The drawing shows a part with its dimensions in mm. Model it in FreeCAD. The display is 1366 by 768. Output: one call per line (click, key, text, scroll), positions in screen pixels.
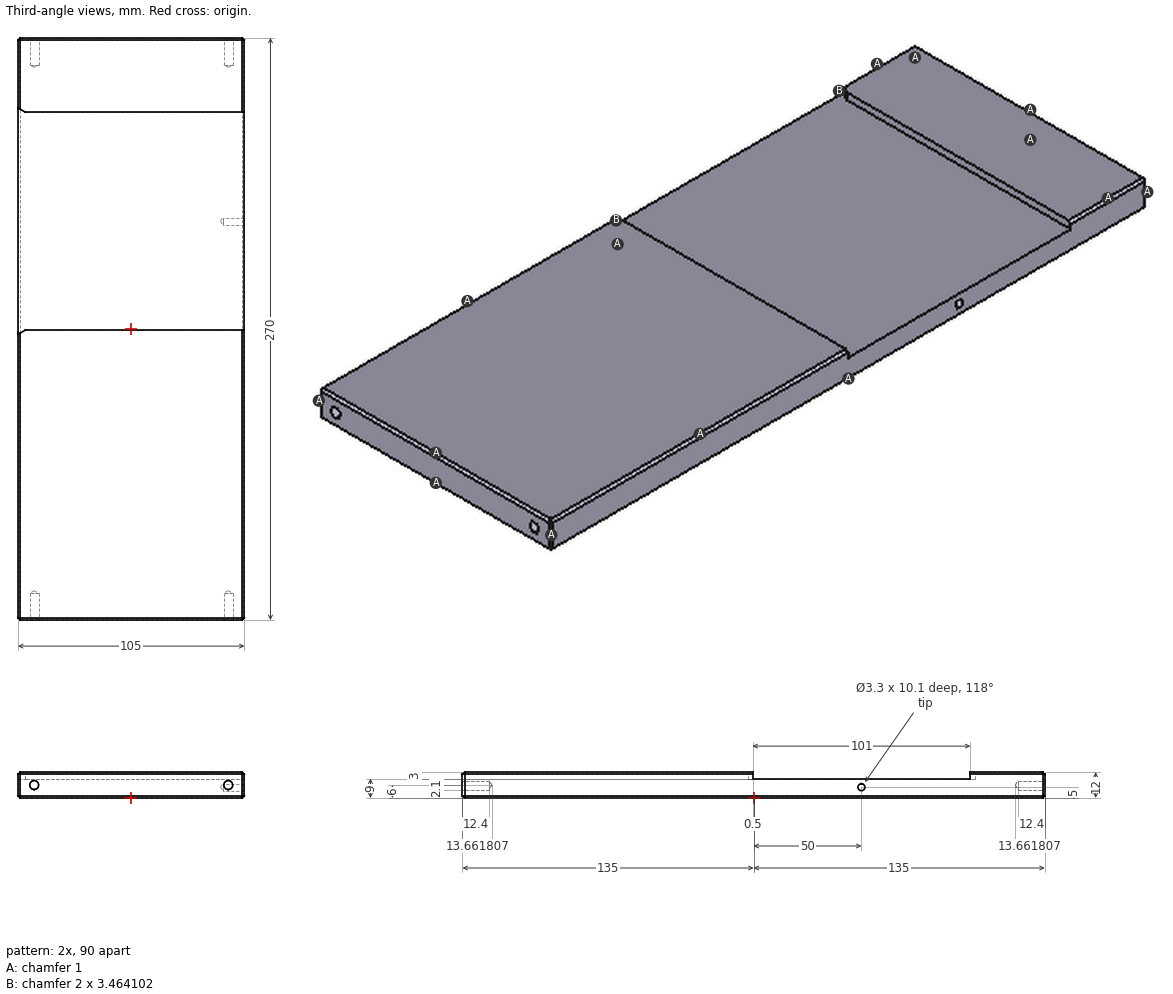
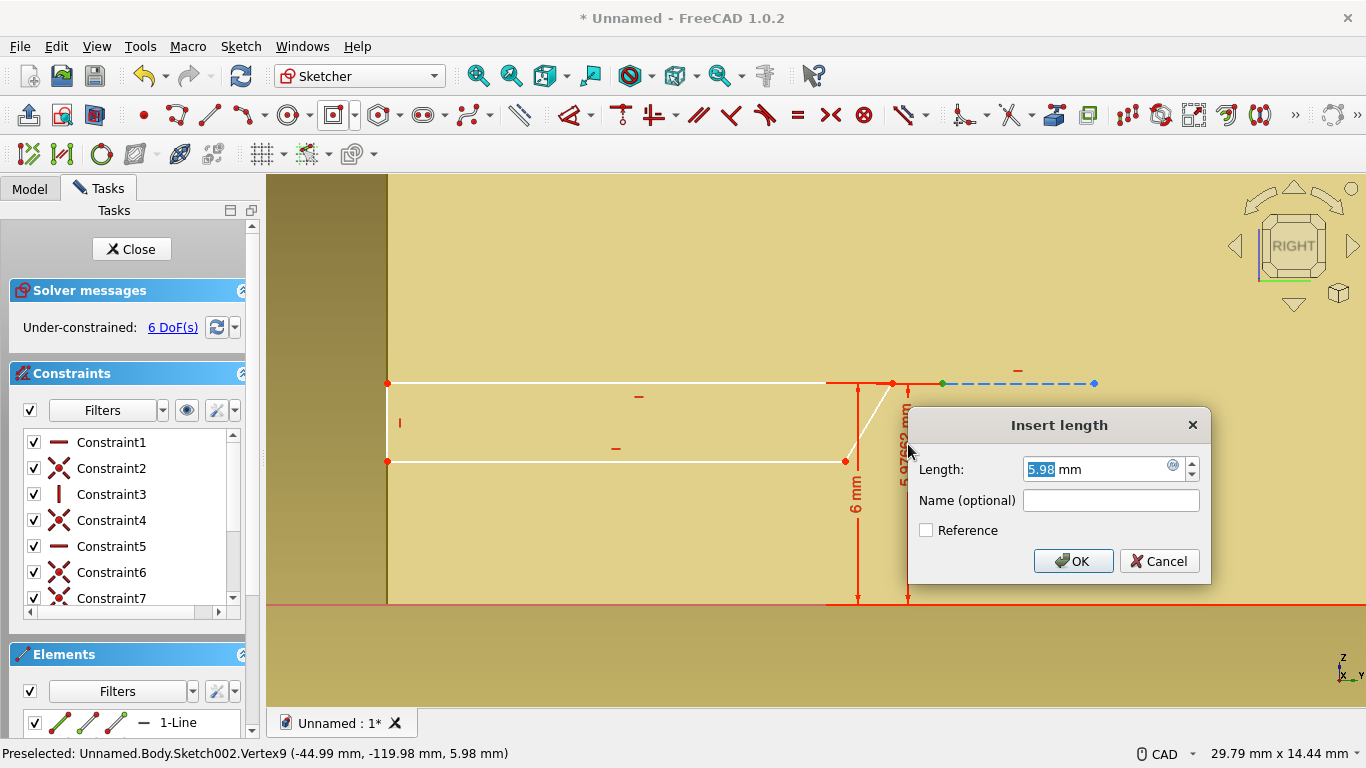
text(6)
key(Return)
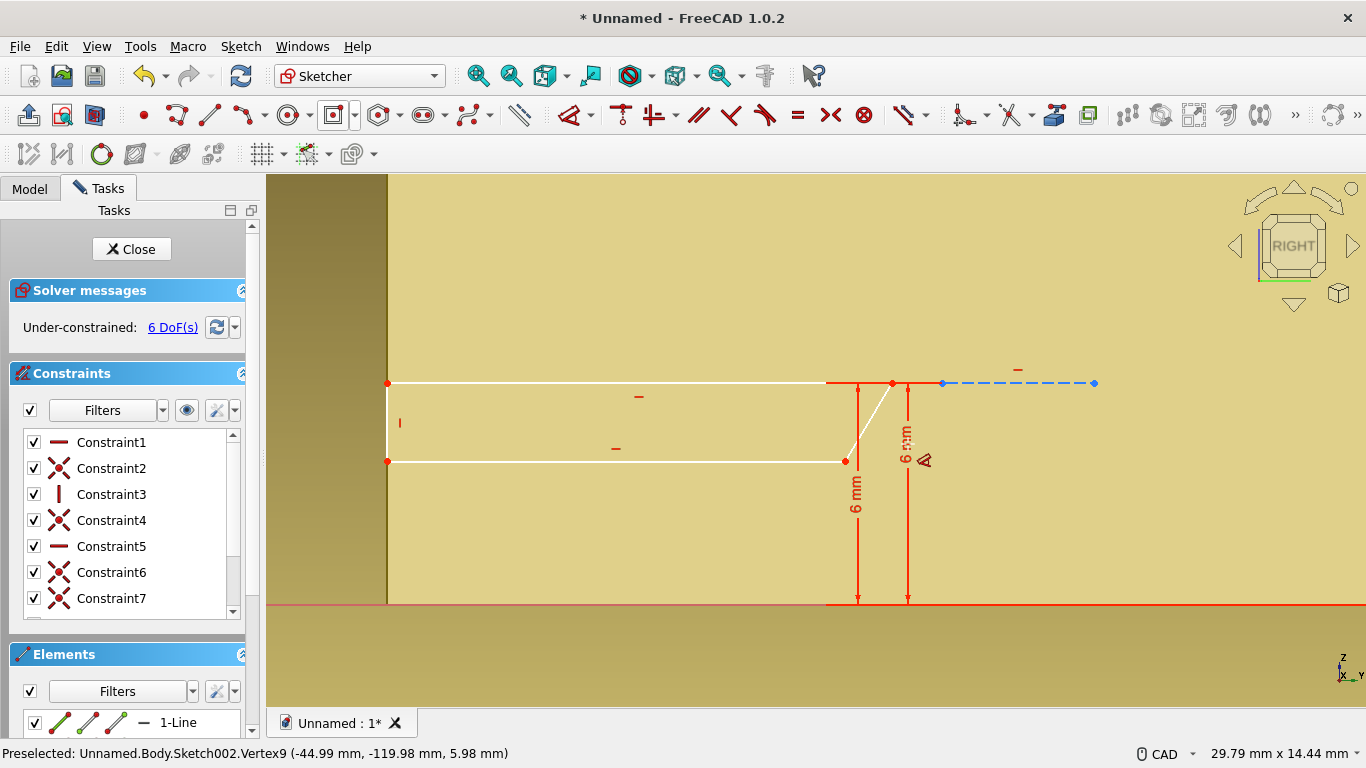
click(387, 407)
click(353, 423)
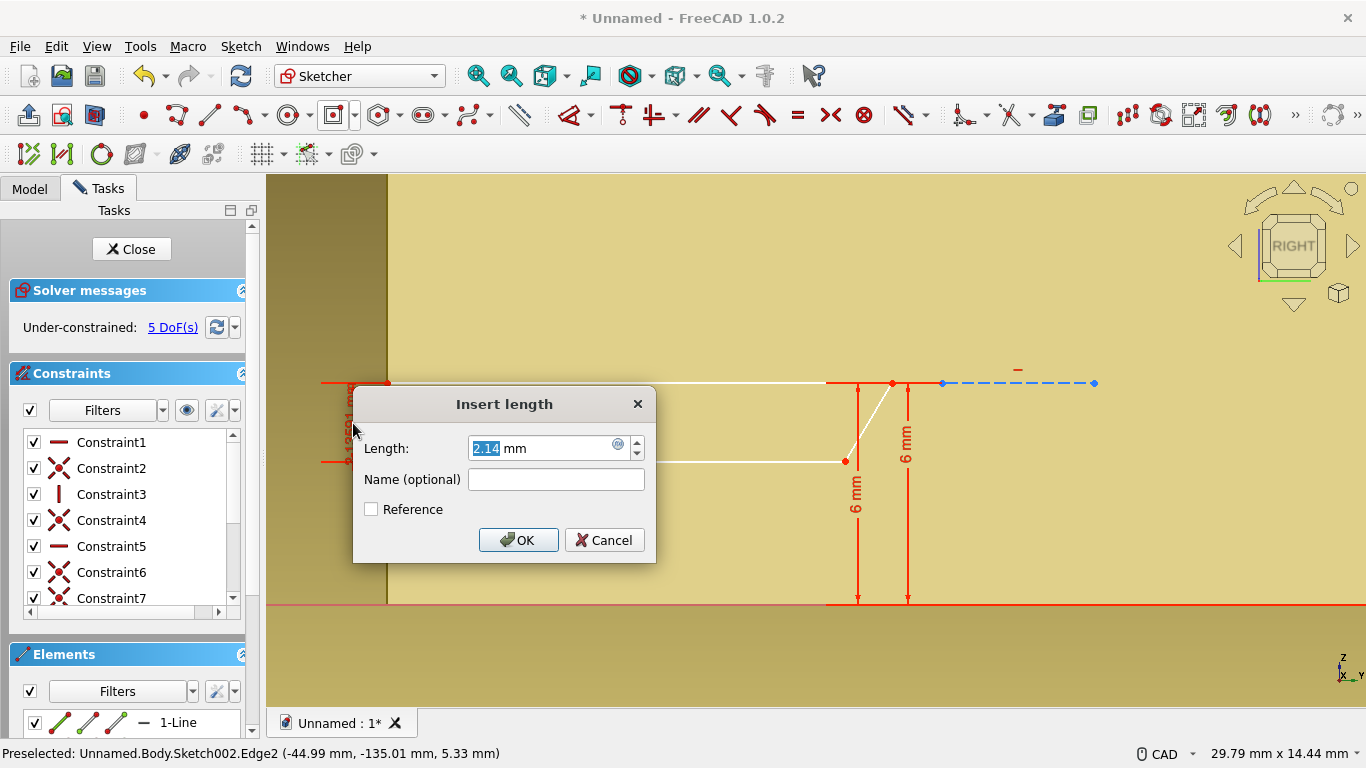
text(2.1)
key(Return)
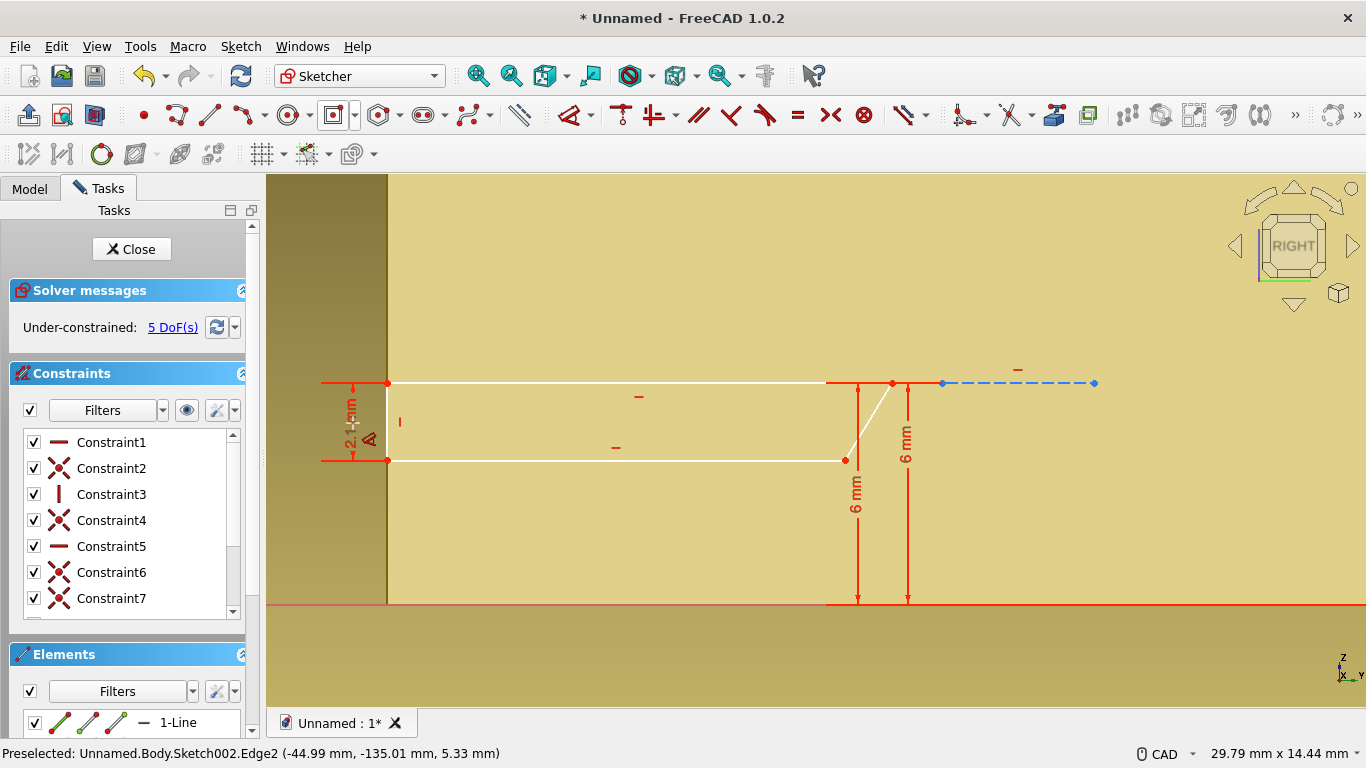
click(524, 461)
click(616, 495)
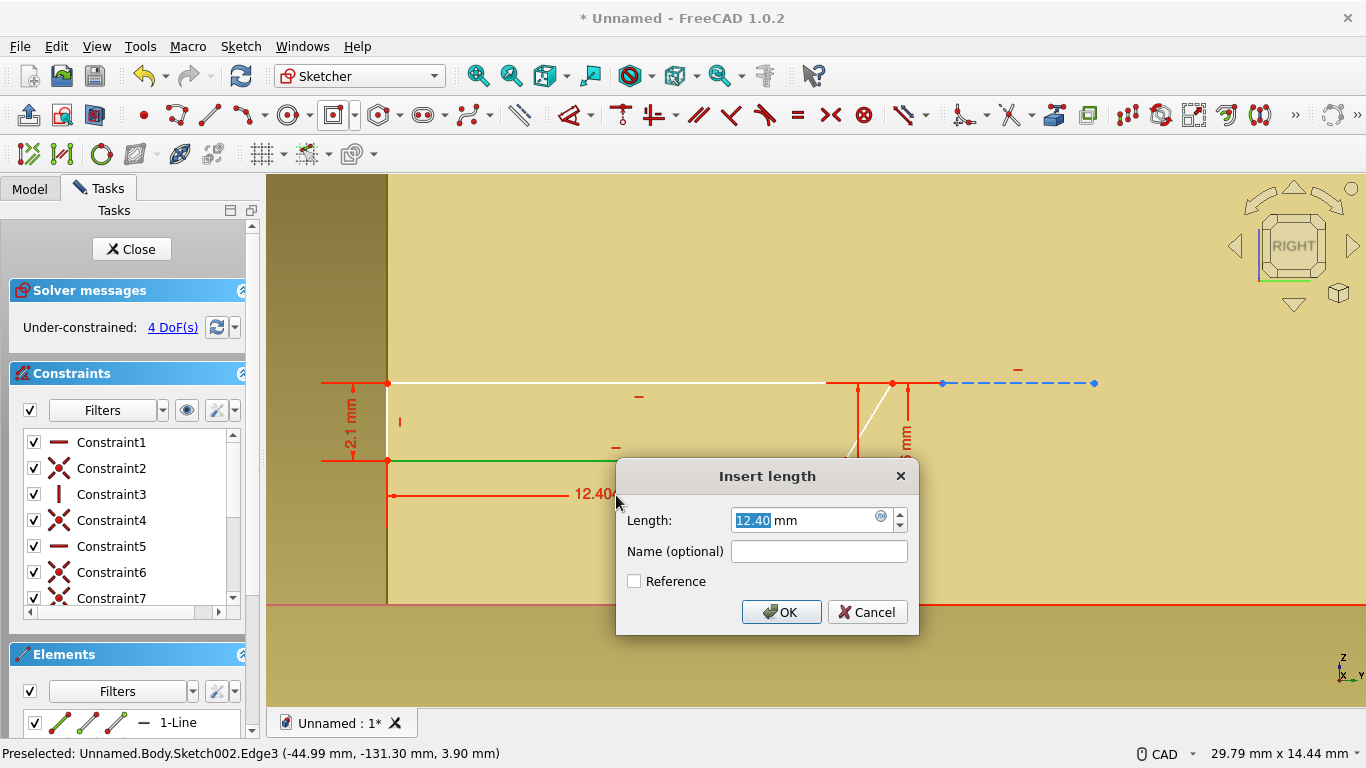
text(12.4)
key(Return)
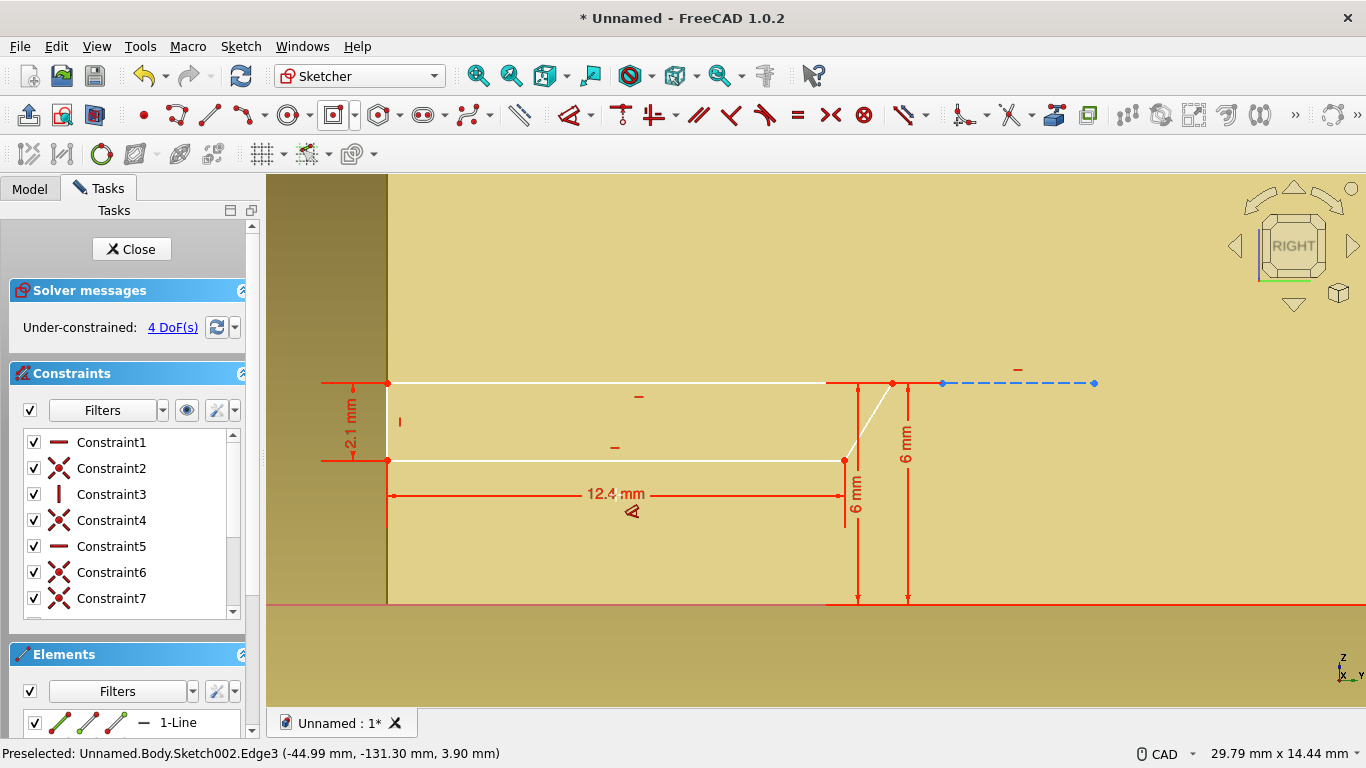
click(387, 383)
click(794, 639)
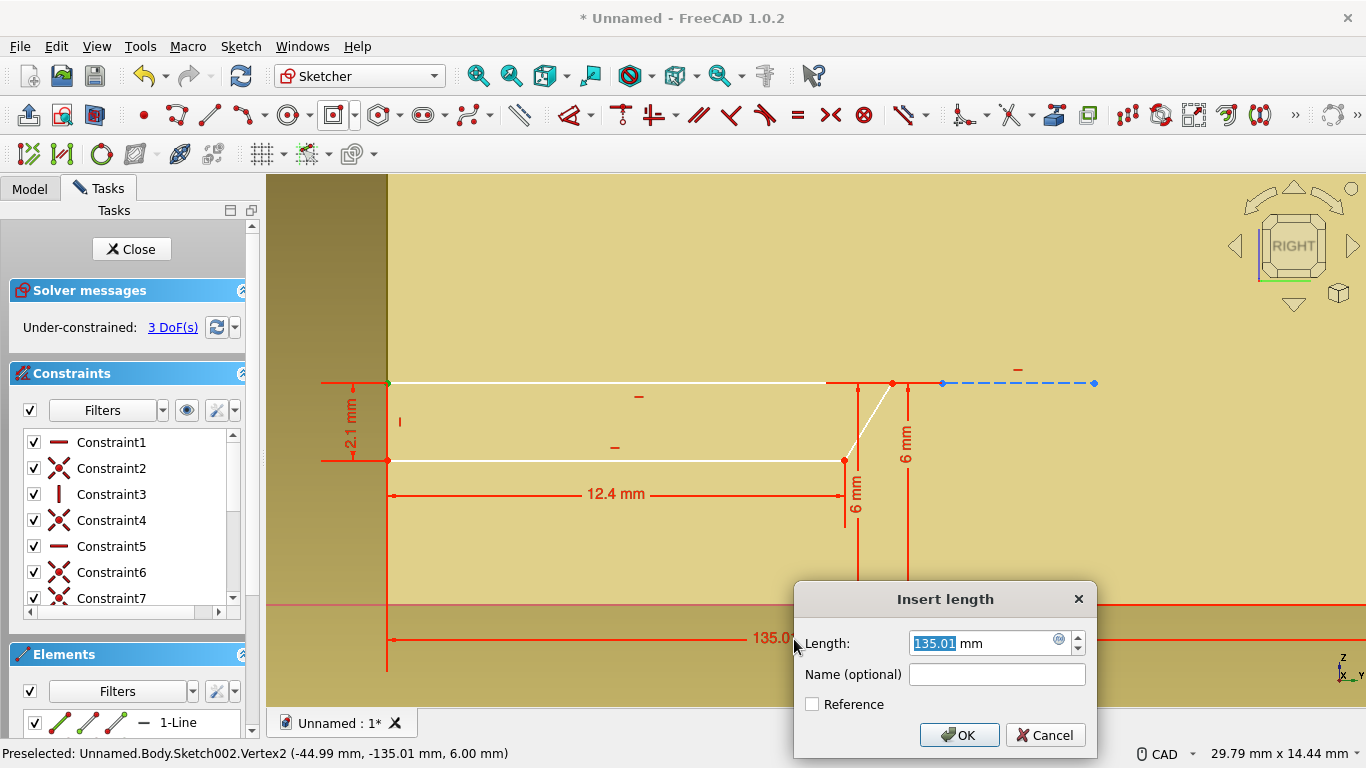
text(135)
key(Return)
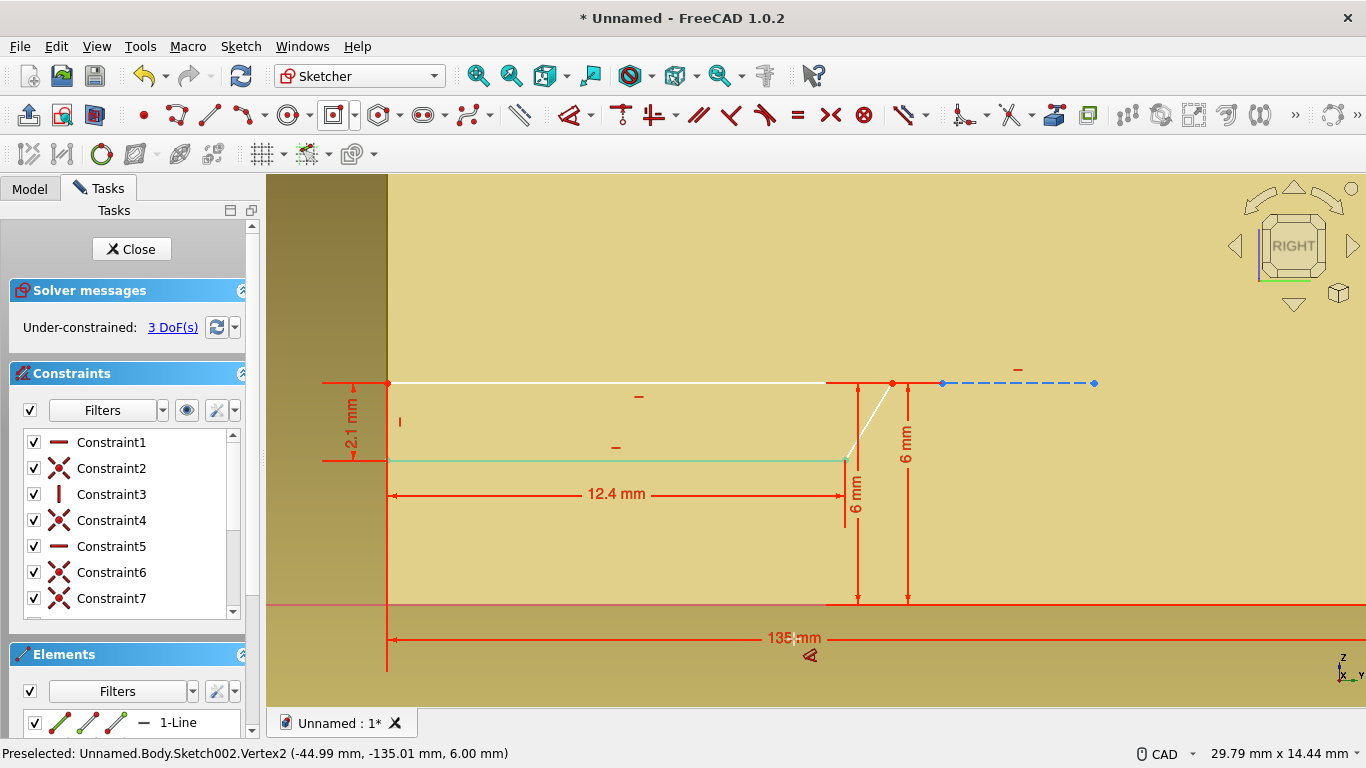
click(741, 383)
click(640, 349)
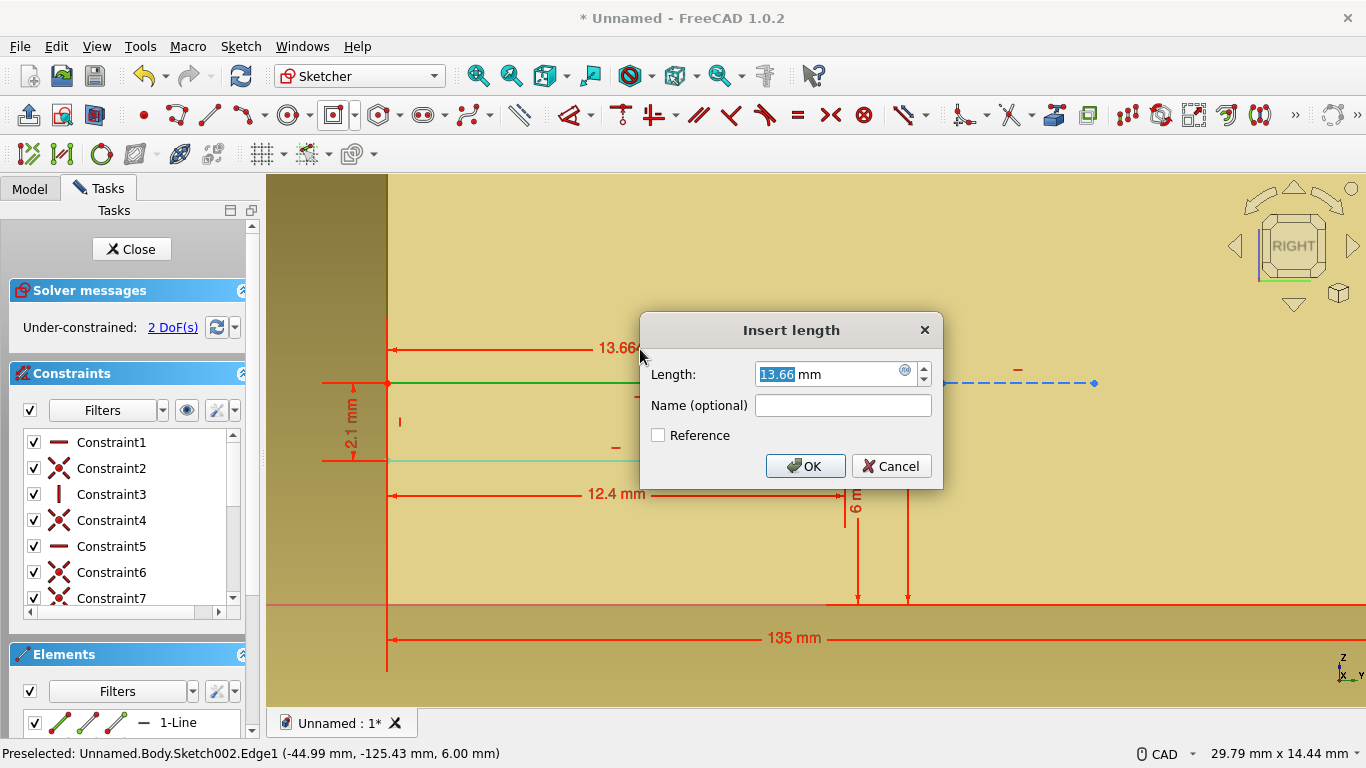
text(13.661807)
key(Return)
key(Escape)